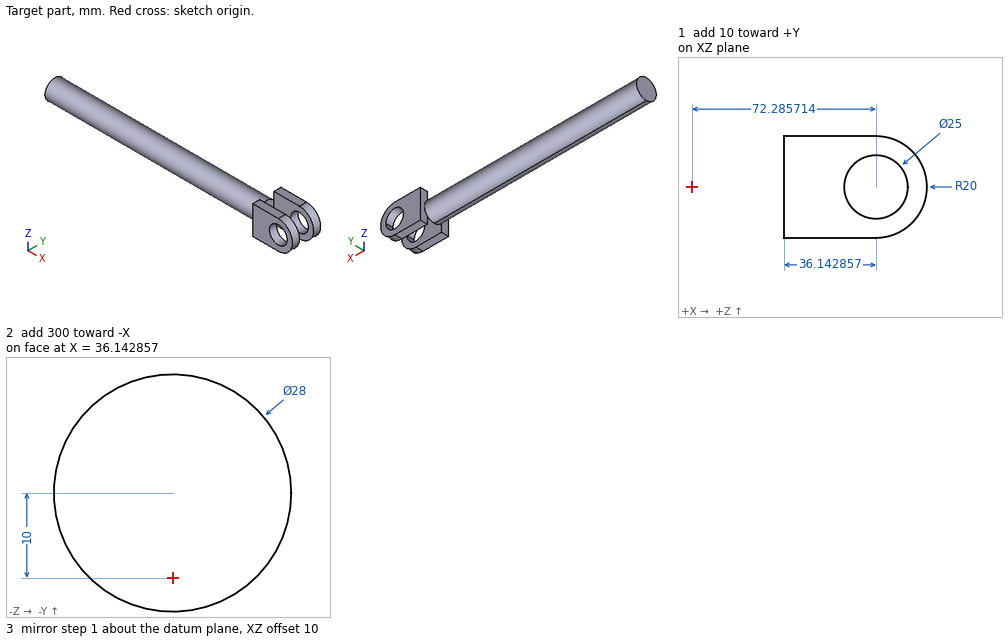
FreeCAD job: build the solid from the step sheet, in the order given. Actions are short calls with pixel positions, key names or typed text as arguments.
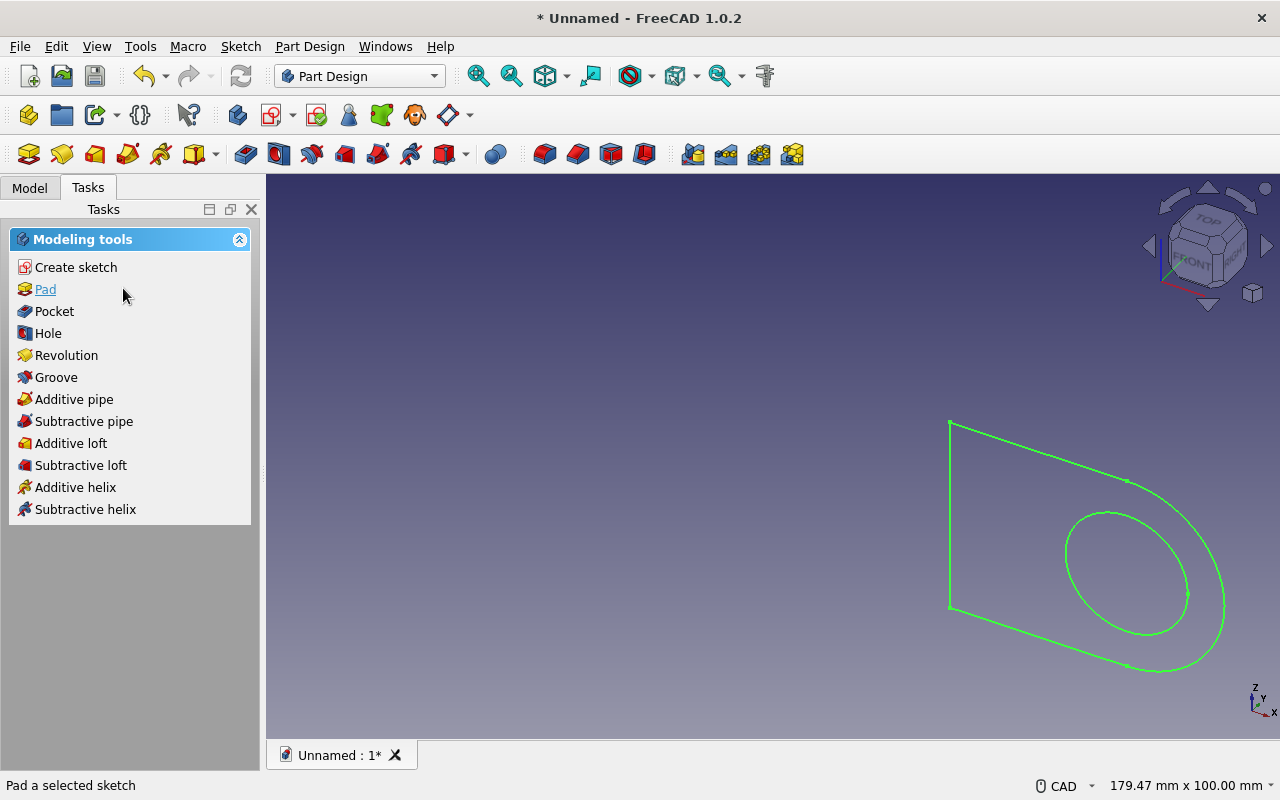
click(29, 154)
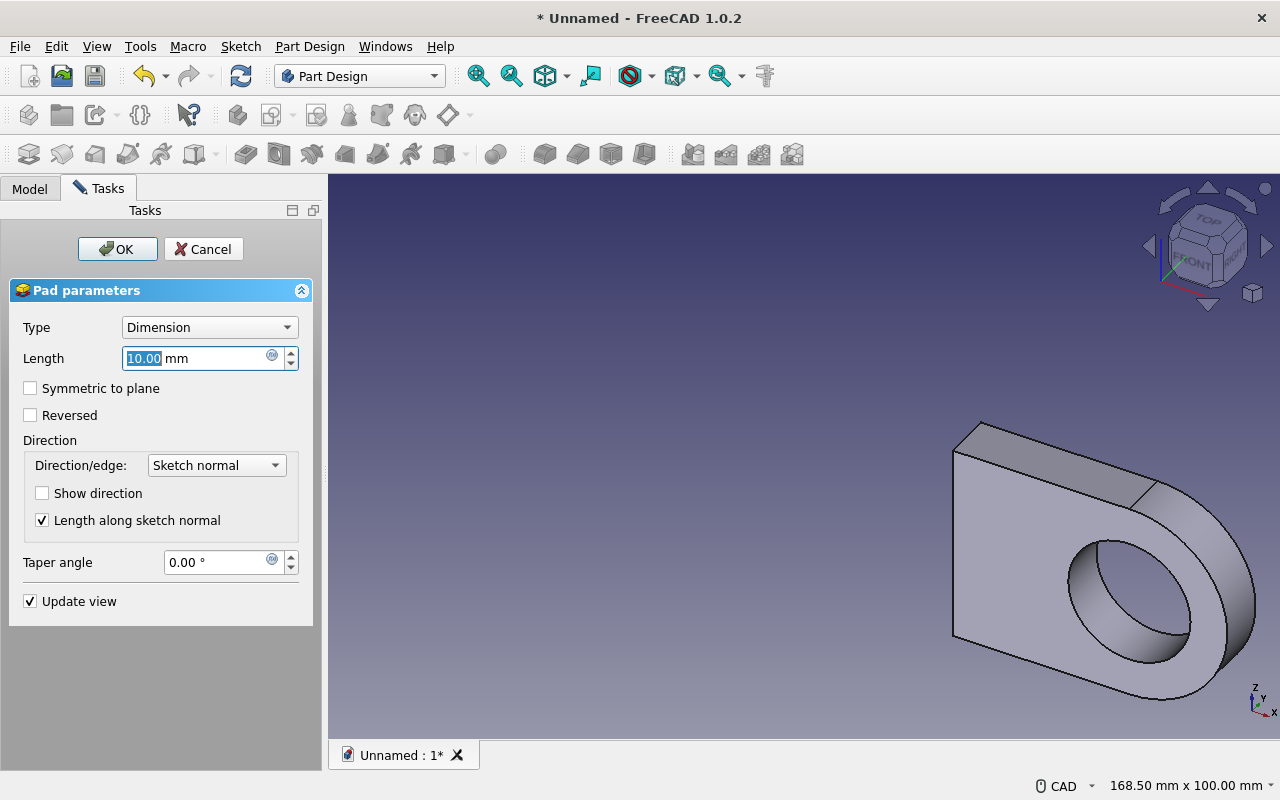
text(10)
key(Tab)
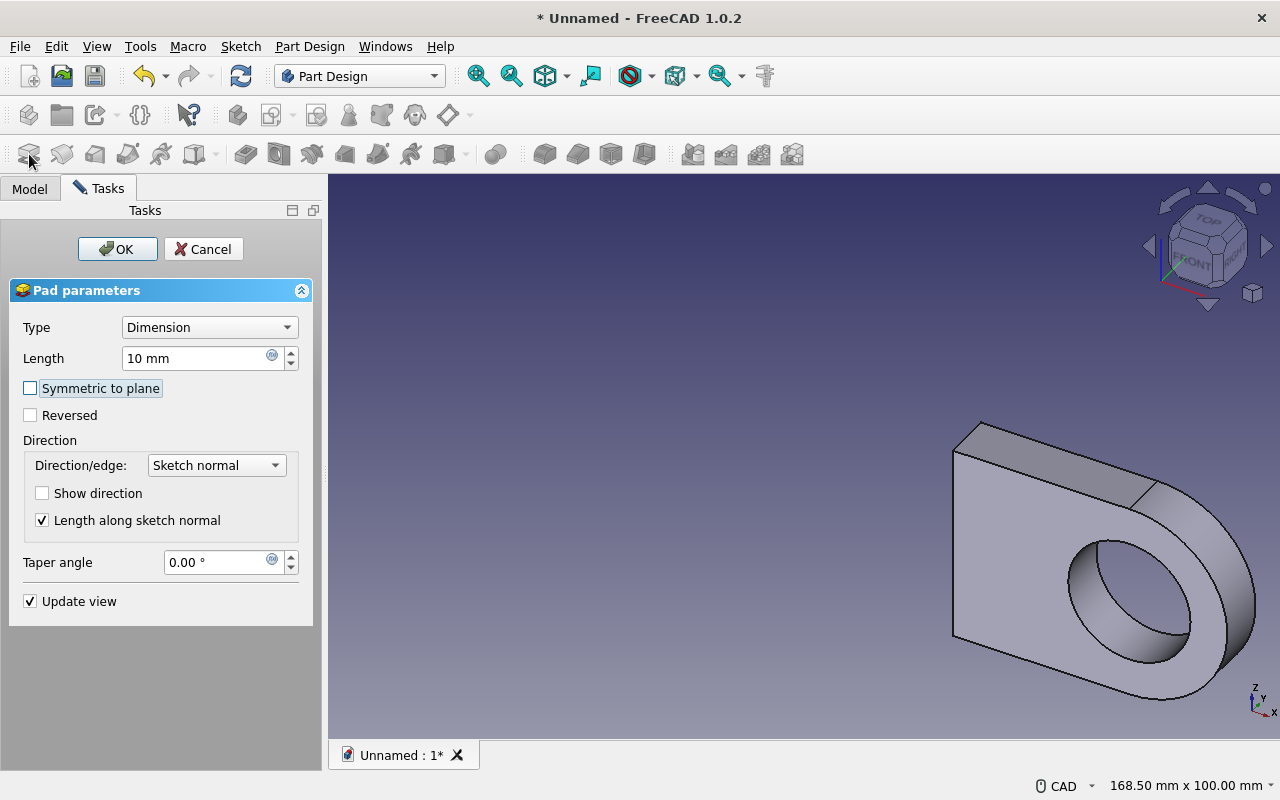
click(31, 415)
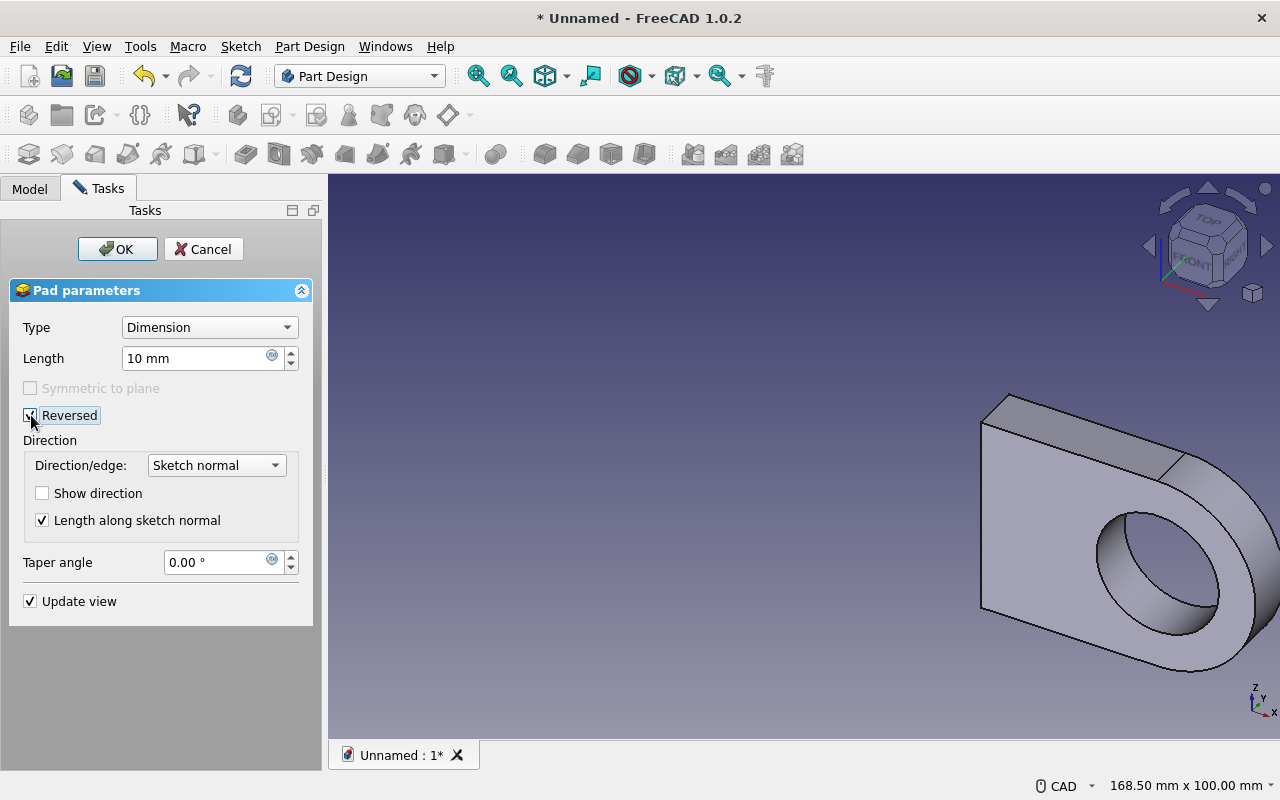
click(118, 249)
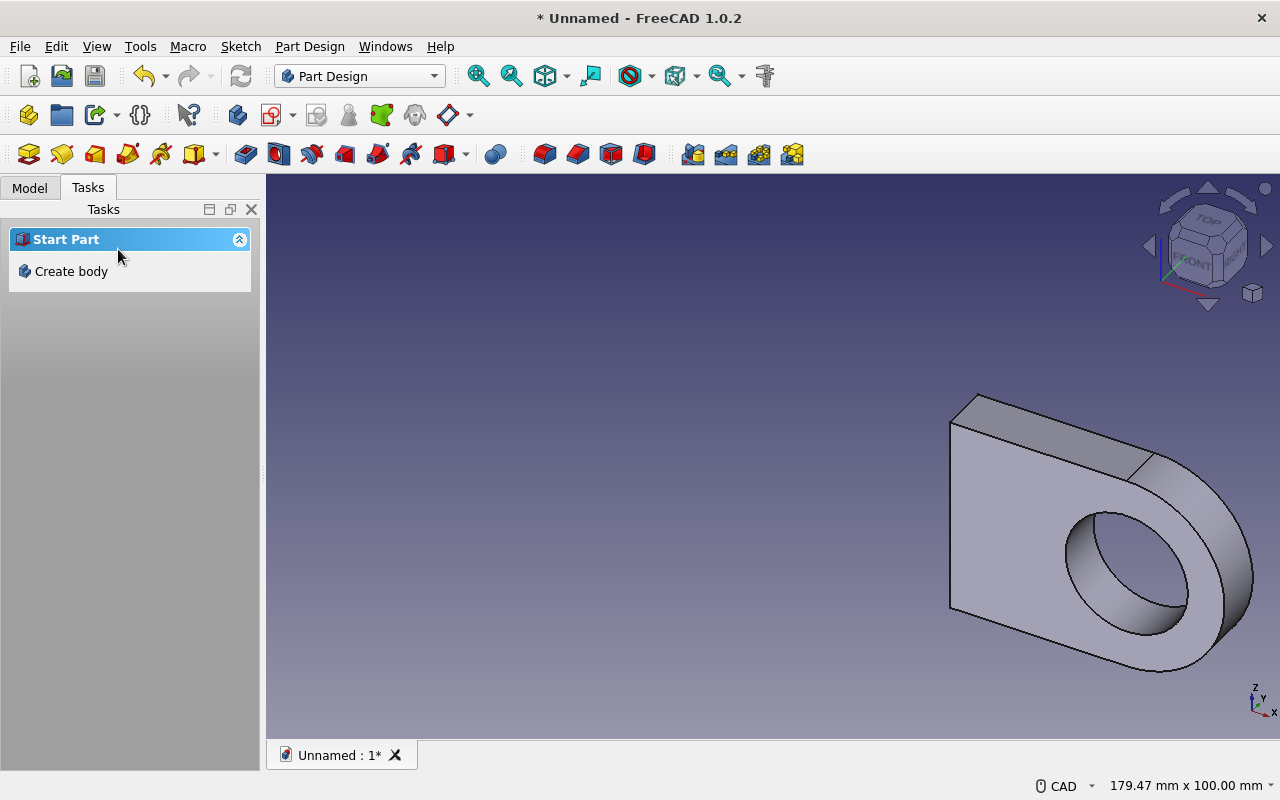
key(6)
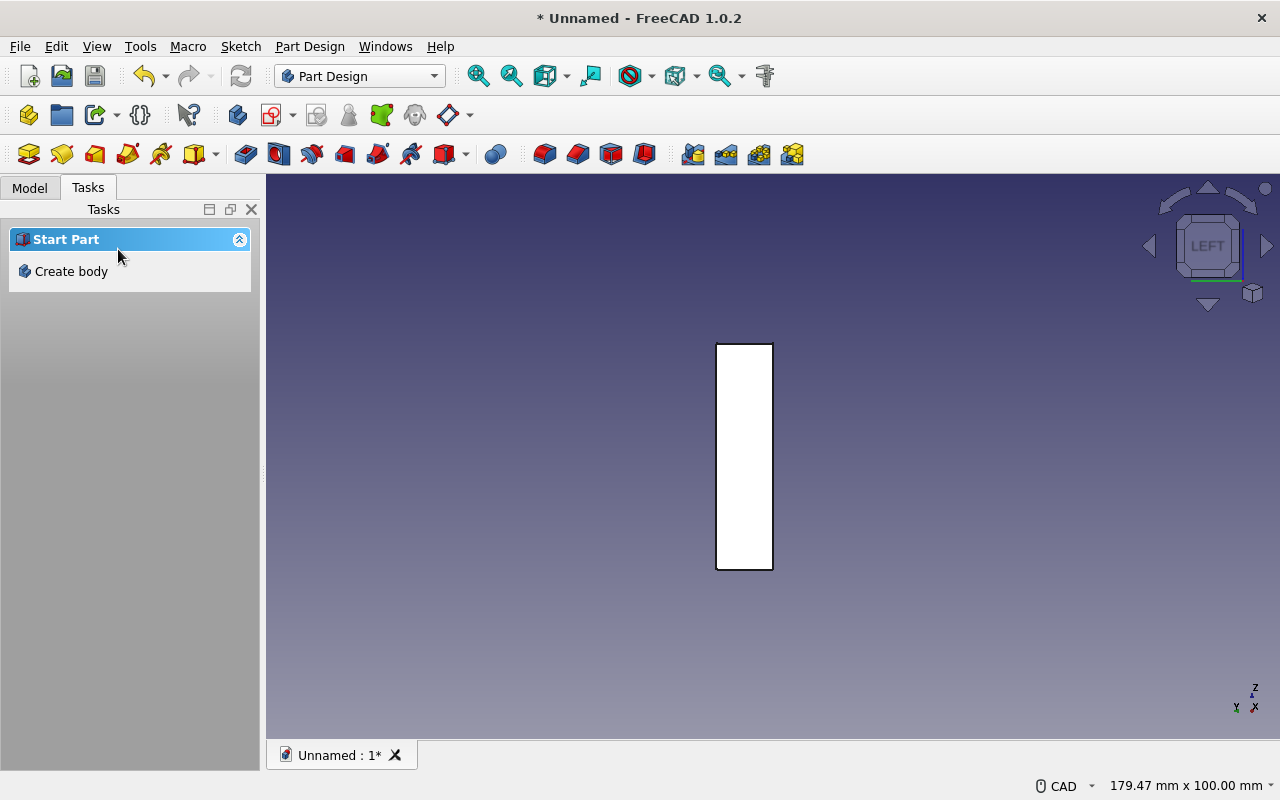
click(479, 76)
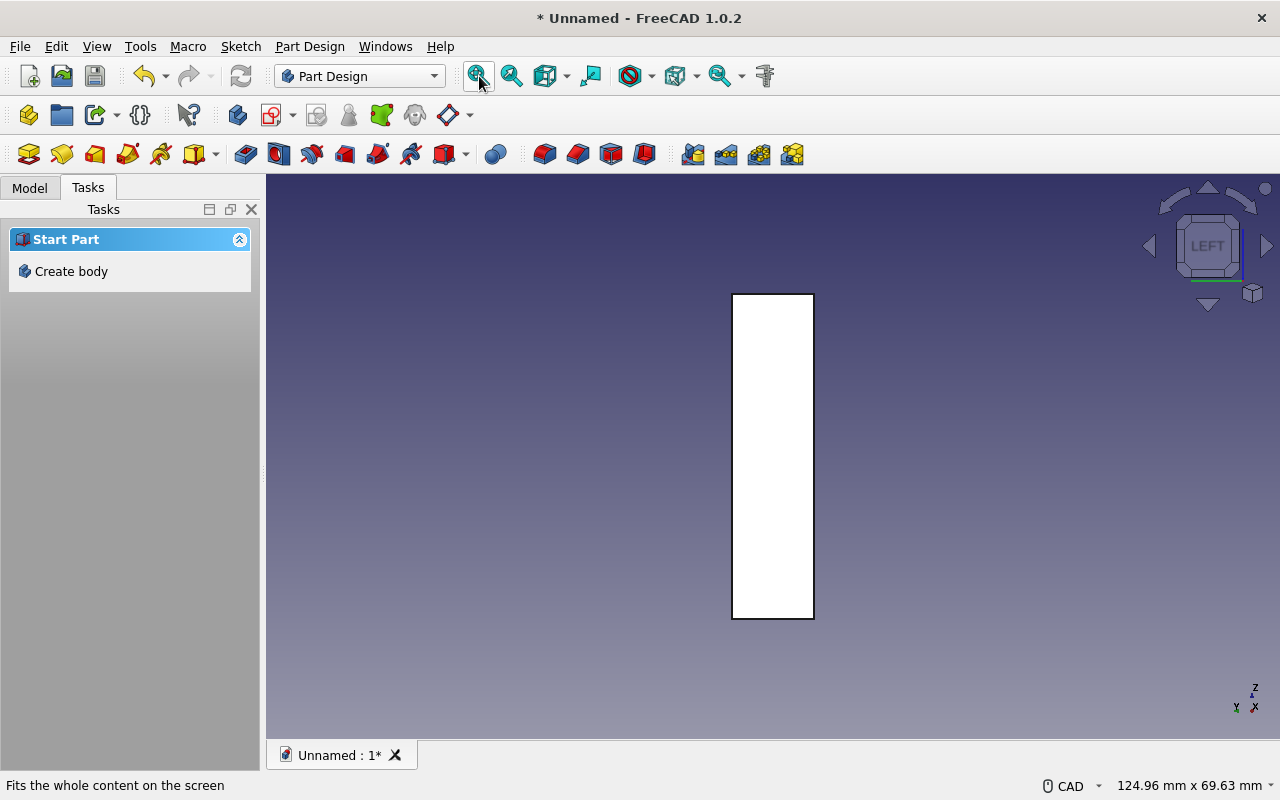
click(773, 455)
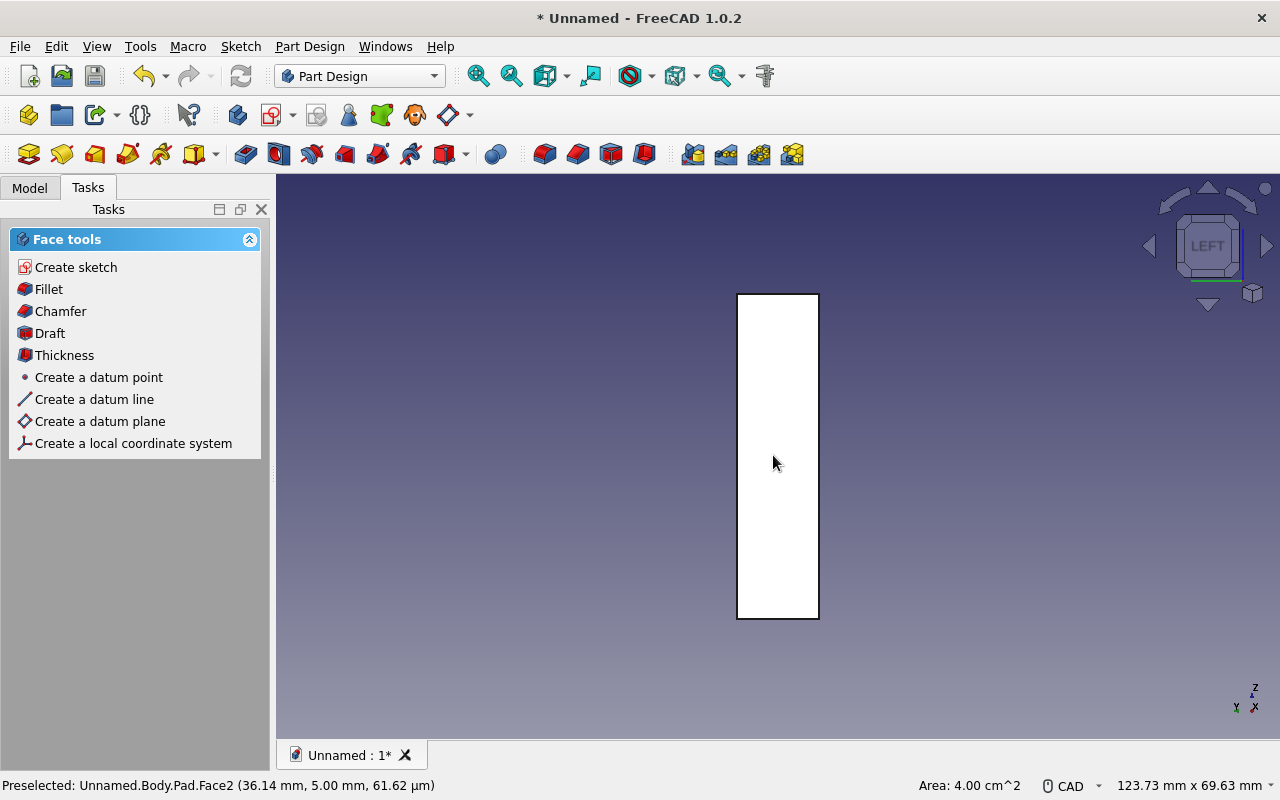
click(270, 116)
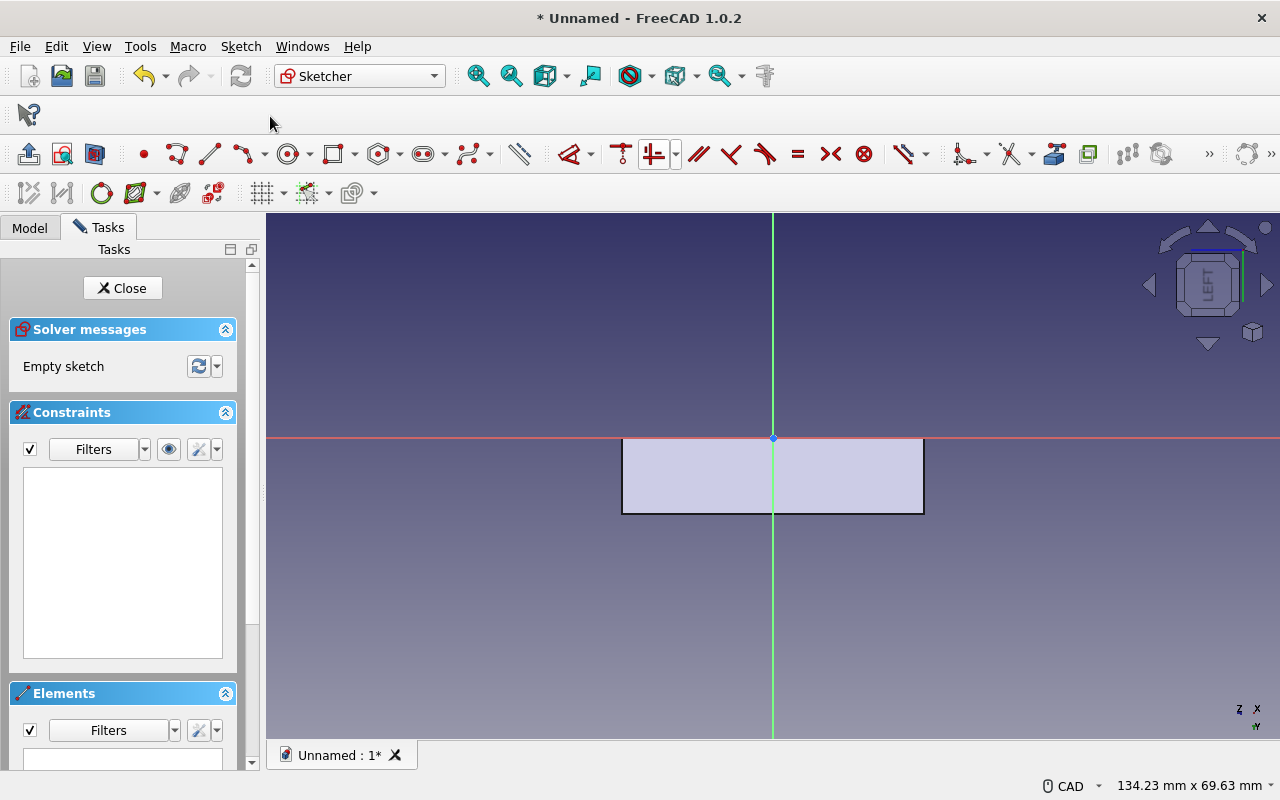
scroll(395, 711, down, 1)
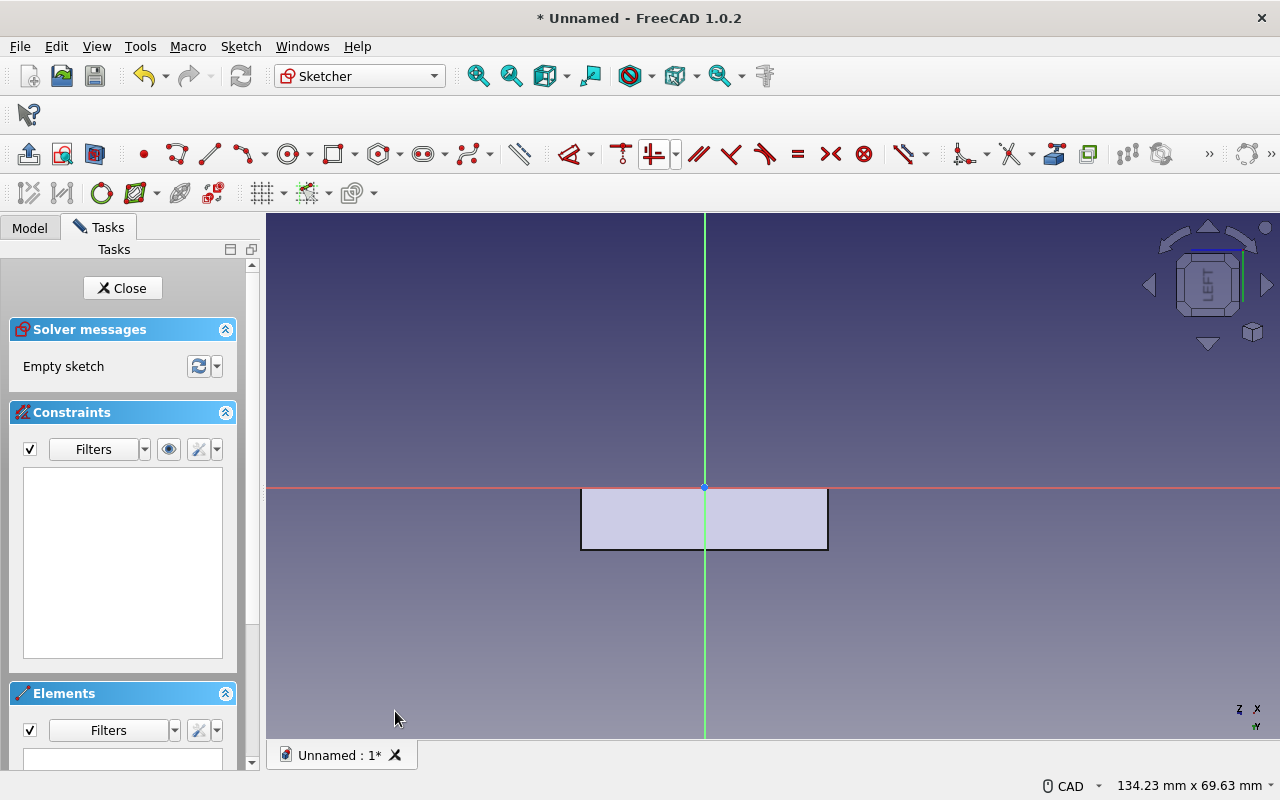
scroll(705, 365, up, 3)